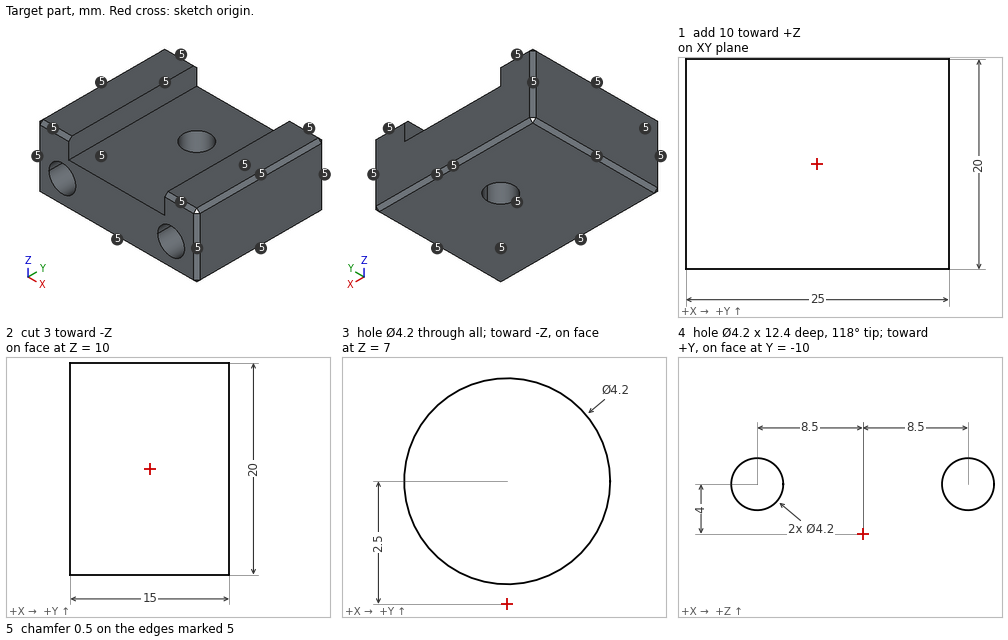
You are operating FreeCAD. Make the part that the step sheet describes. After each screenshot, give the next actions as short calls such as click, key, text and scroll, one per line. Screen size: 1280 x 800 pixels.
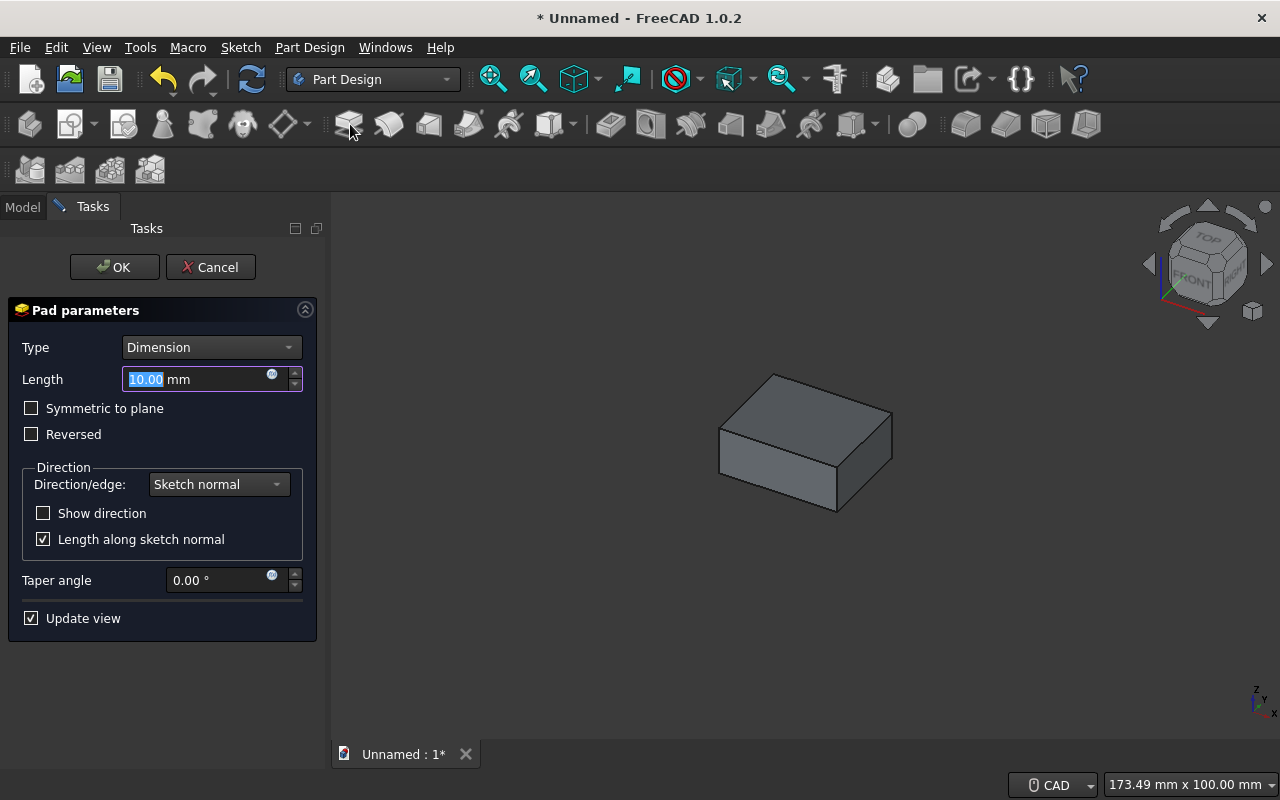
text(10)
key(Tab)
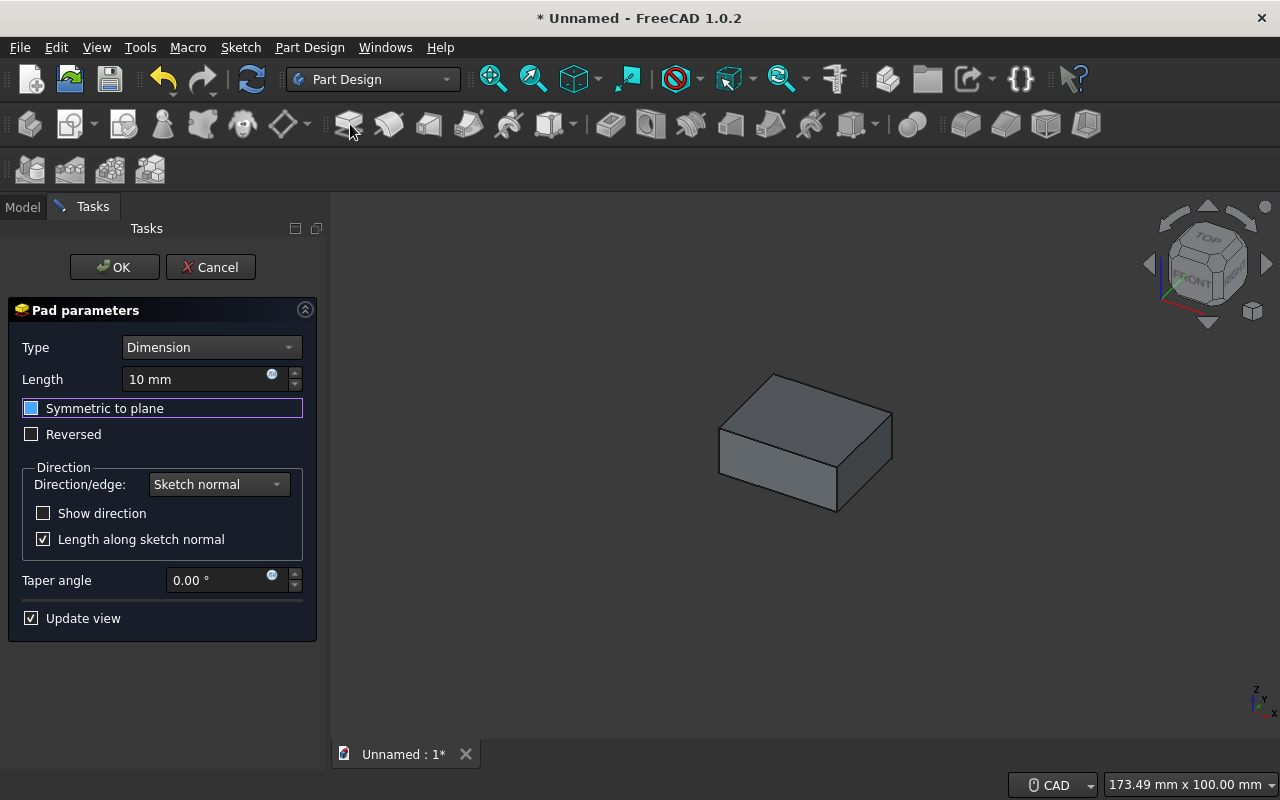
click(115, 267)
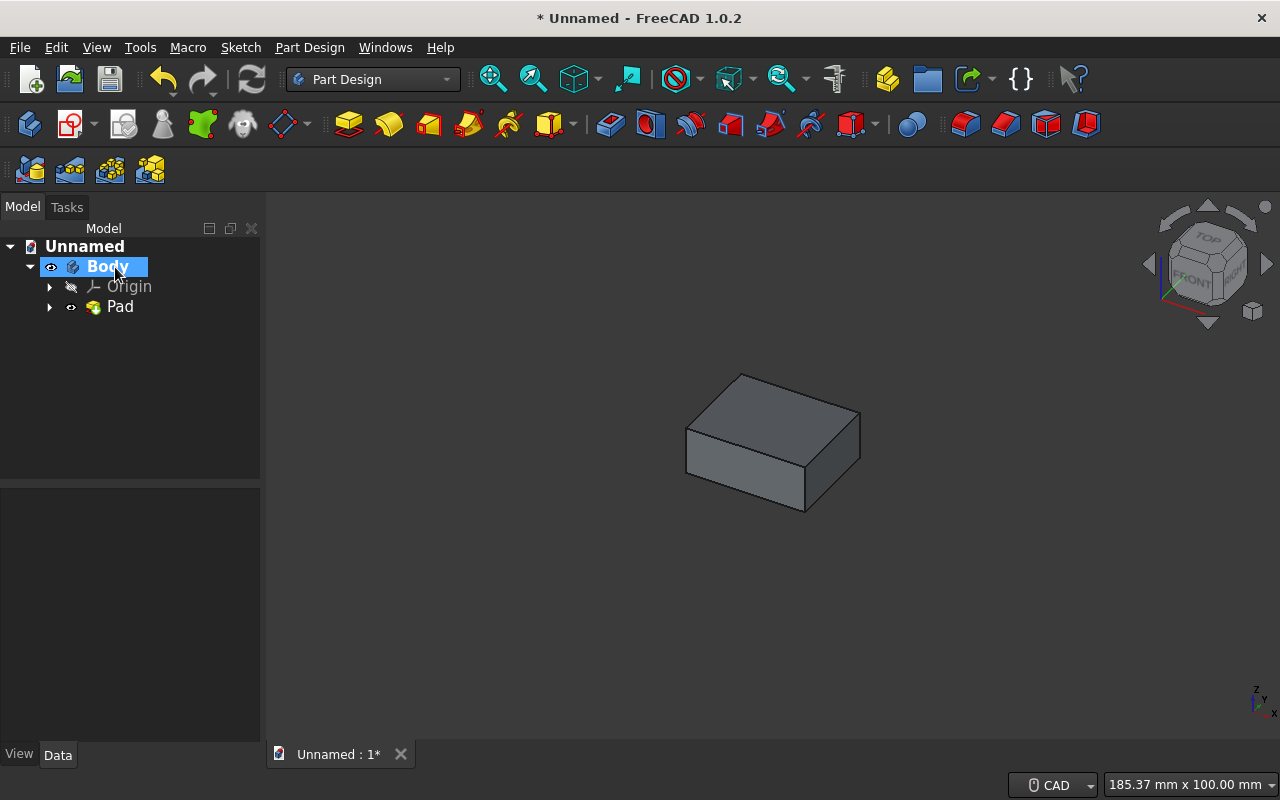
key(v)
key(f)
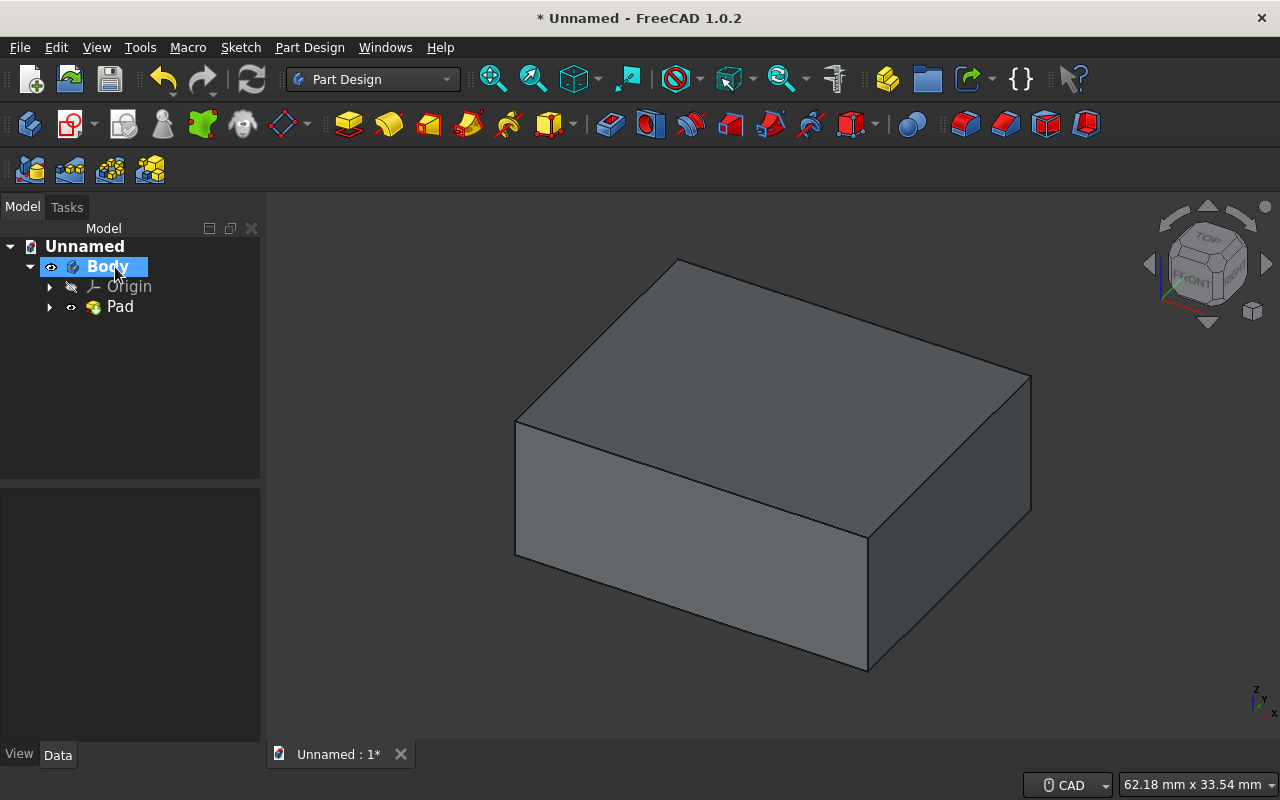
click(773, 398)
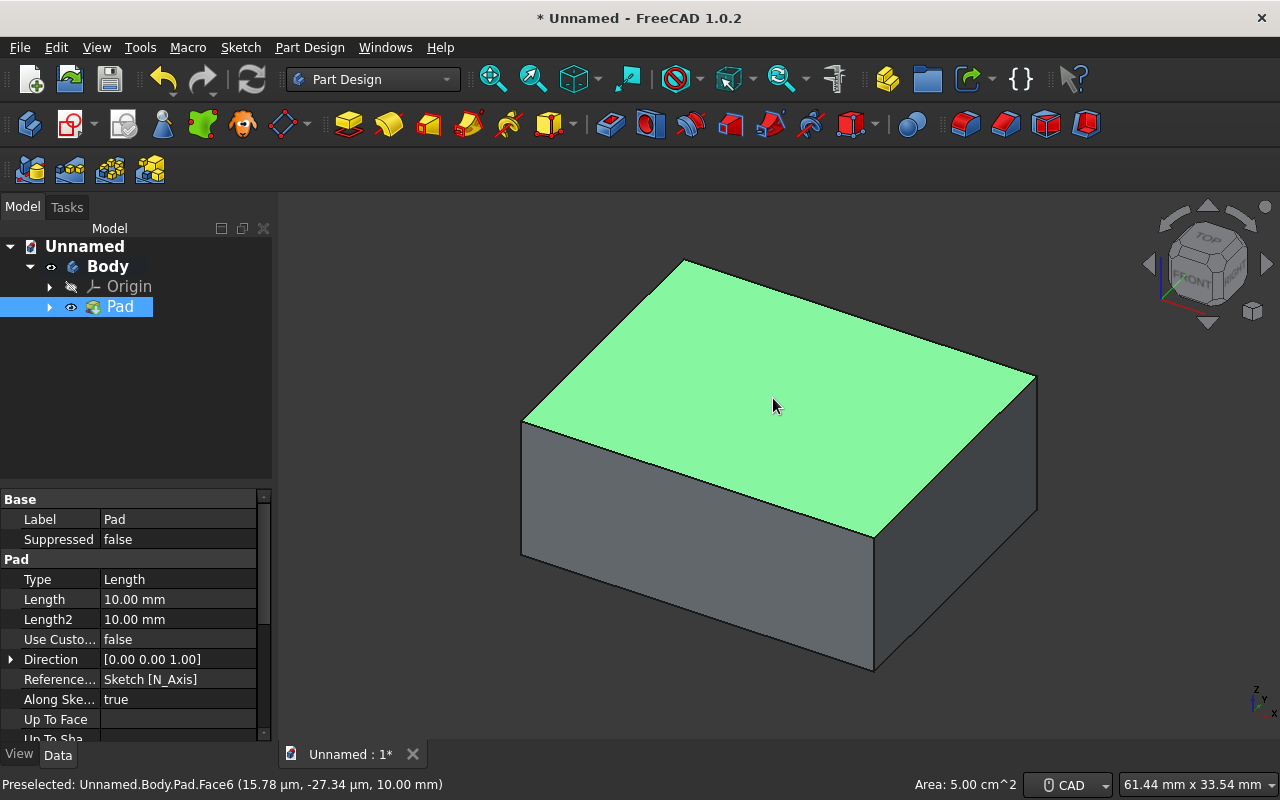
click(70, 124)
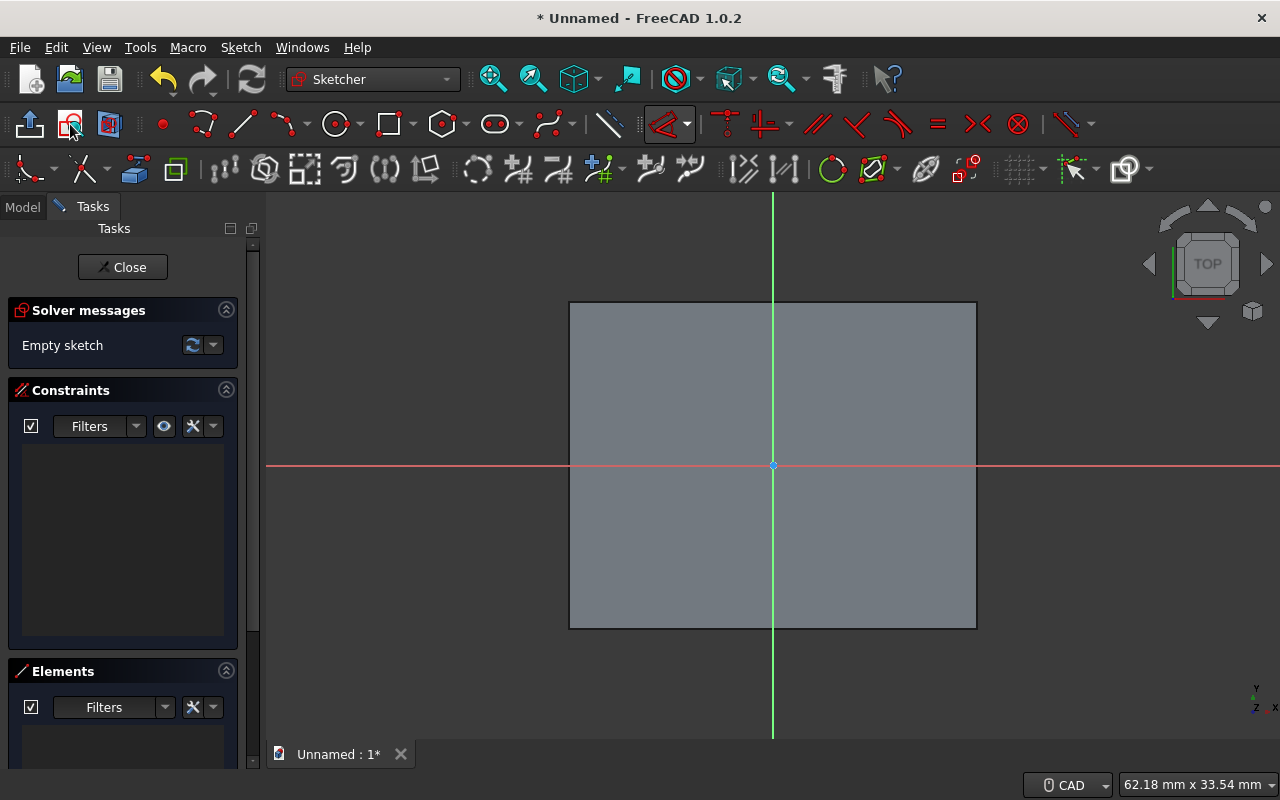
key(g)
key(v)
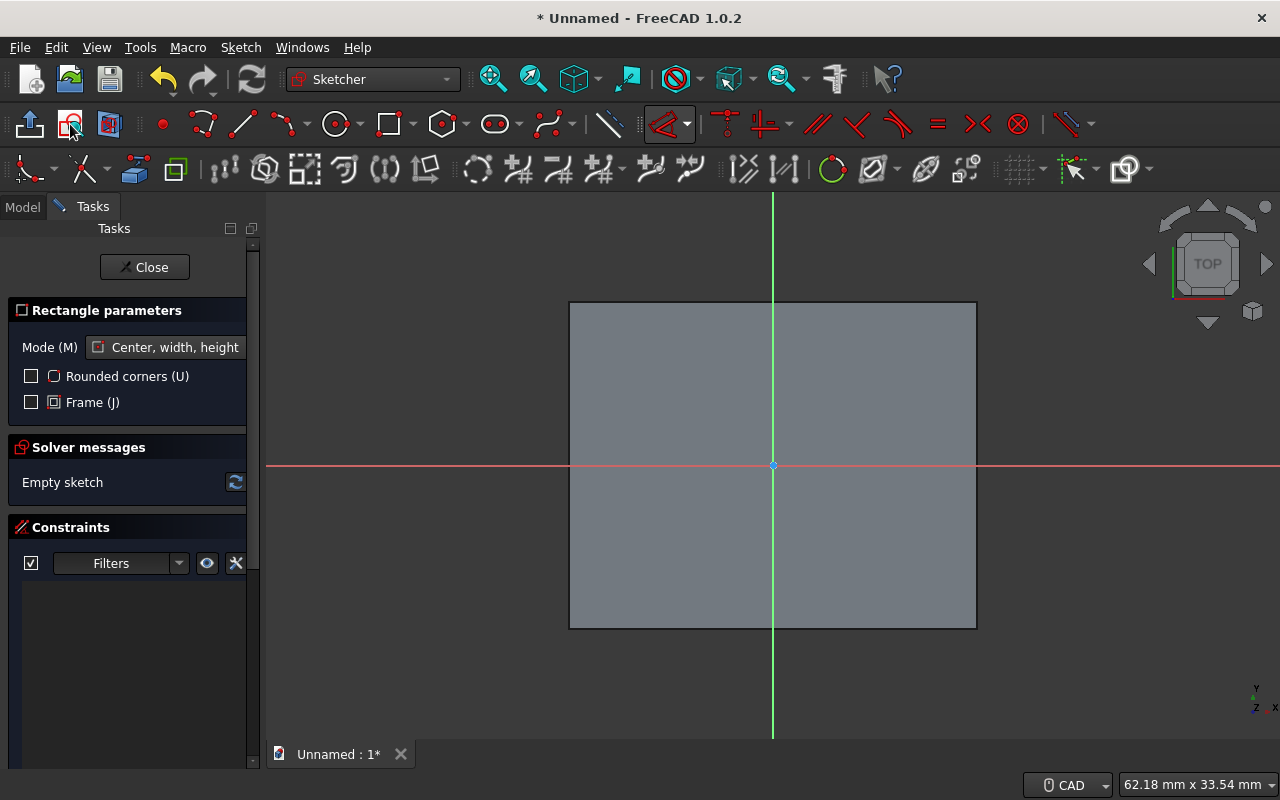
click(773, 466)
move(895, 302)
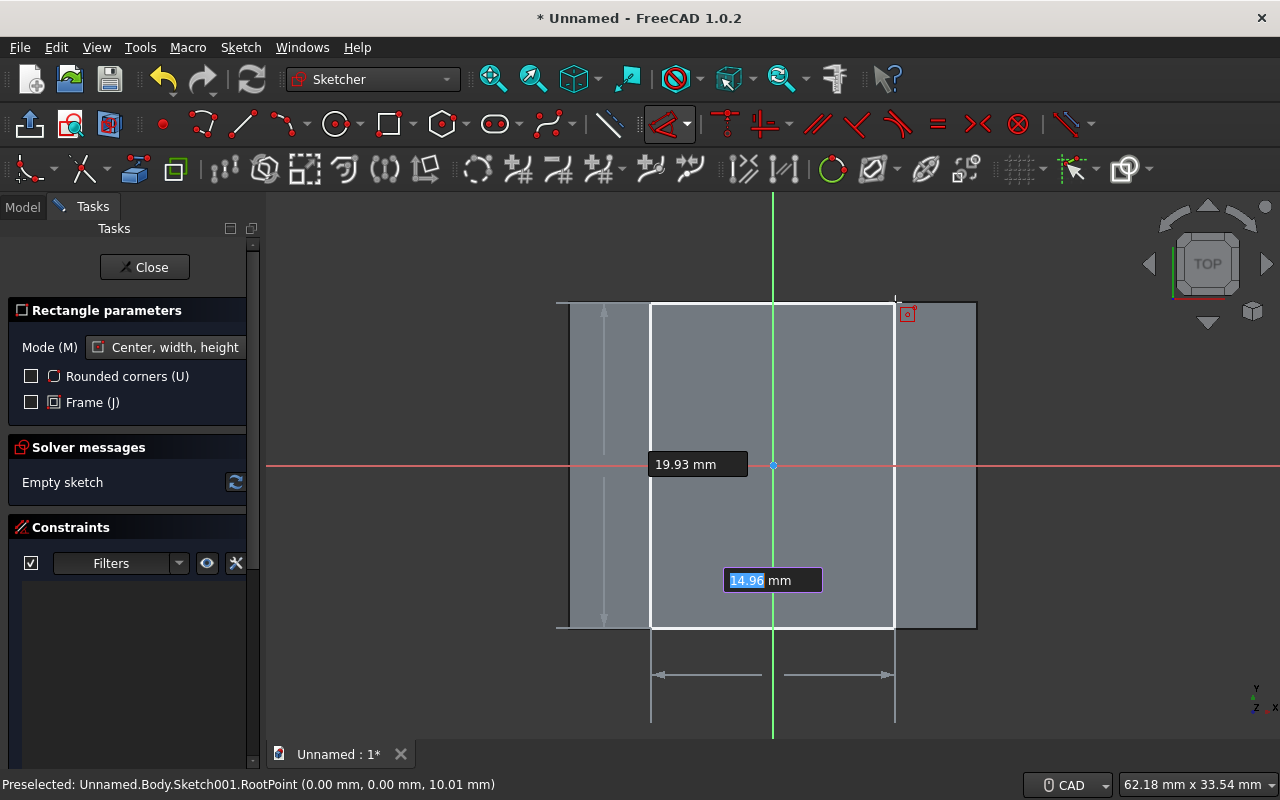
text(15)
key(Tab)
text(20)
key(Return)
key(Escape)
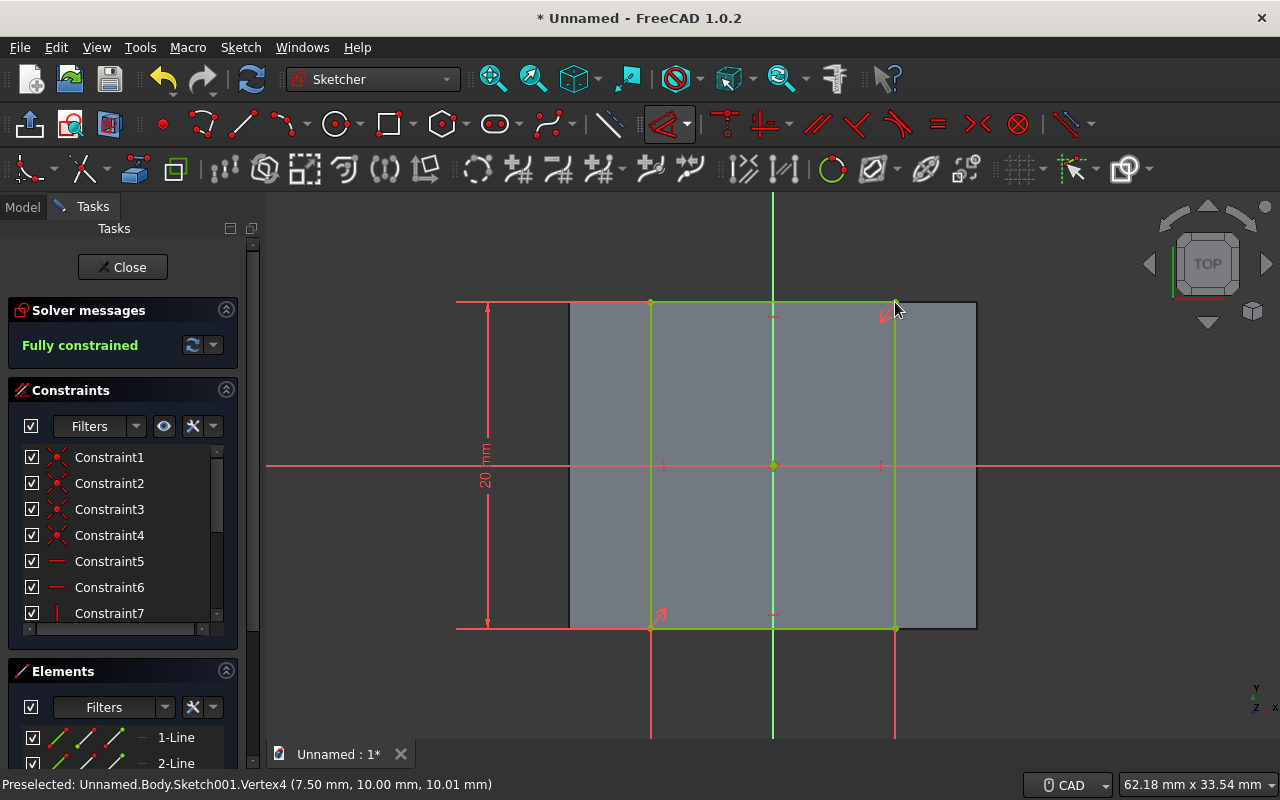
click(123, 267)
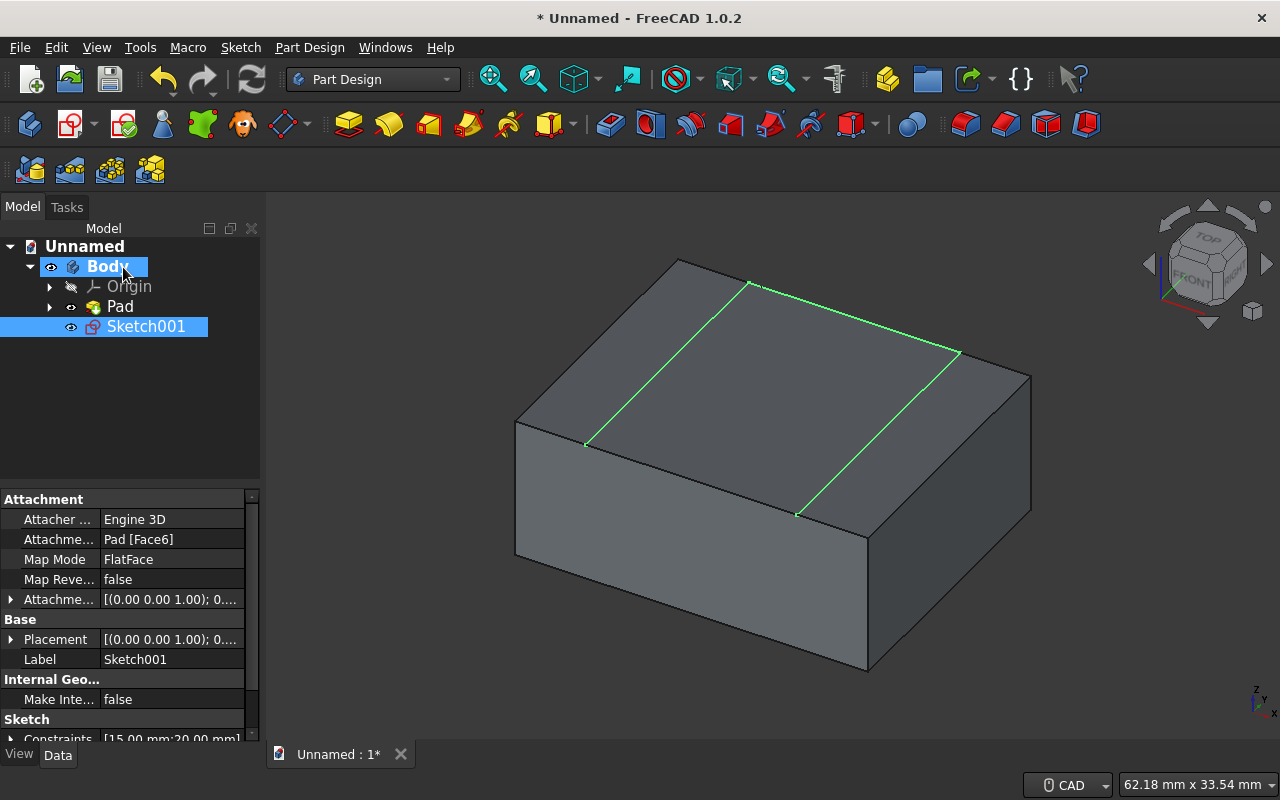
click(612, 124)